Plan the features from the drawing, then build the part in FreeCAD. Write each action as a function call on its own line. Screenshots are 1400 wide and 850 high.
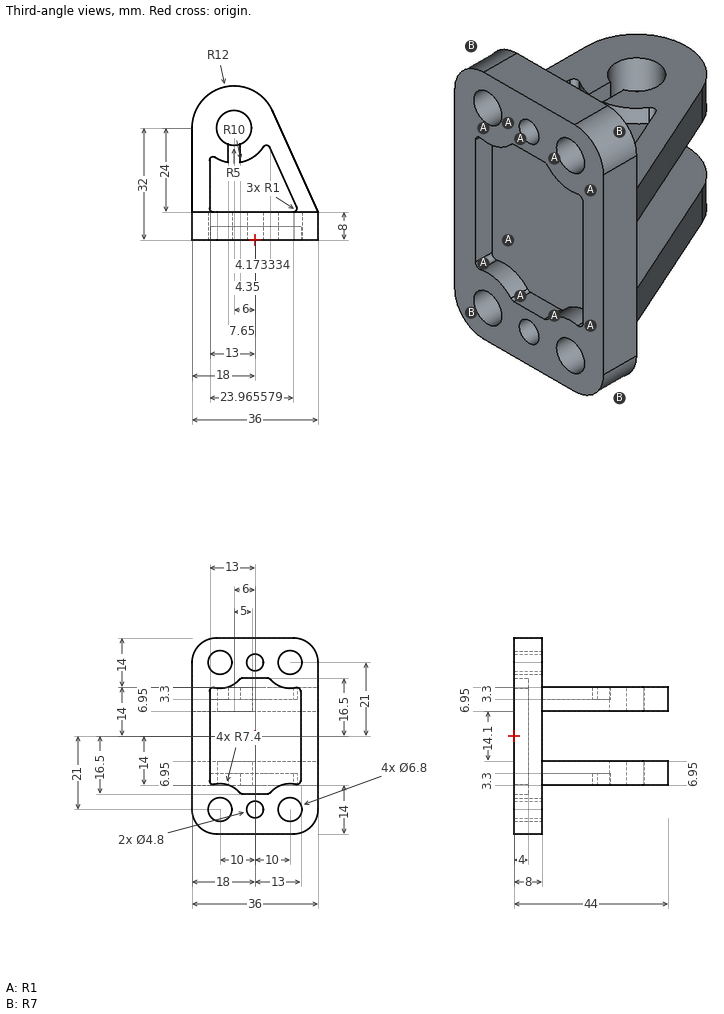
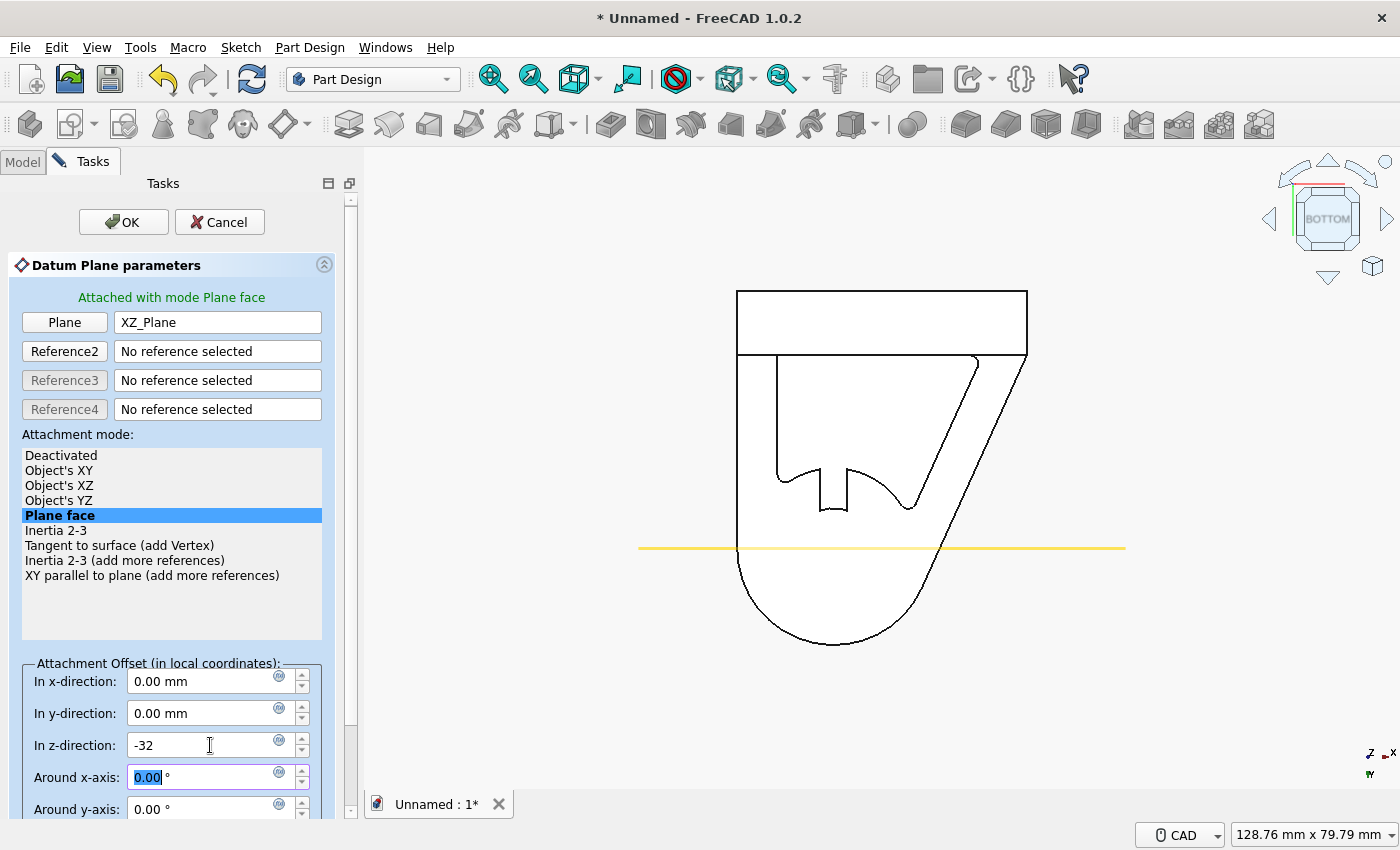
click(124, 222)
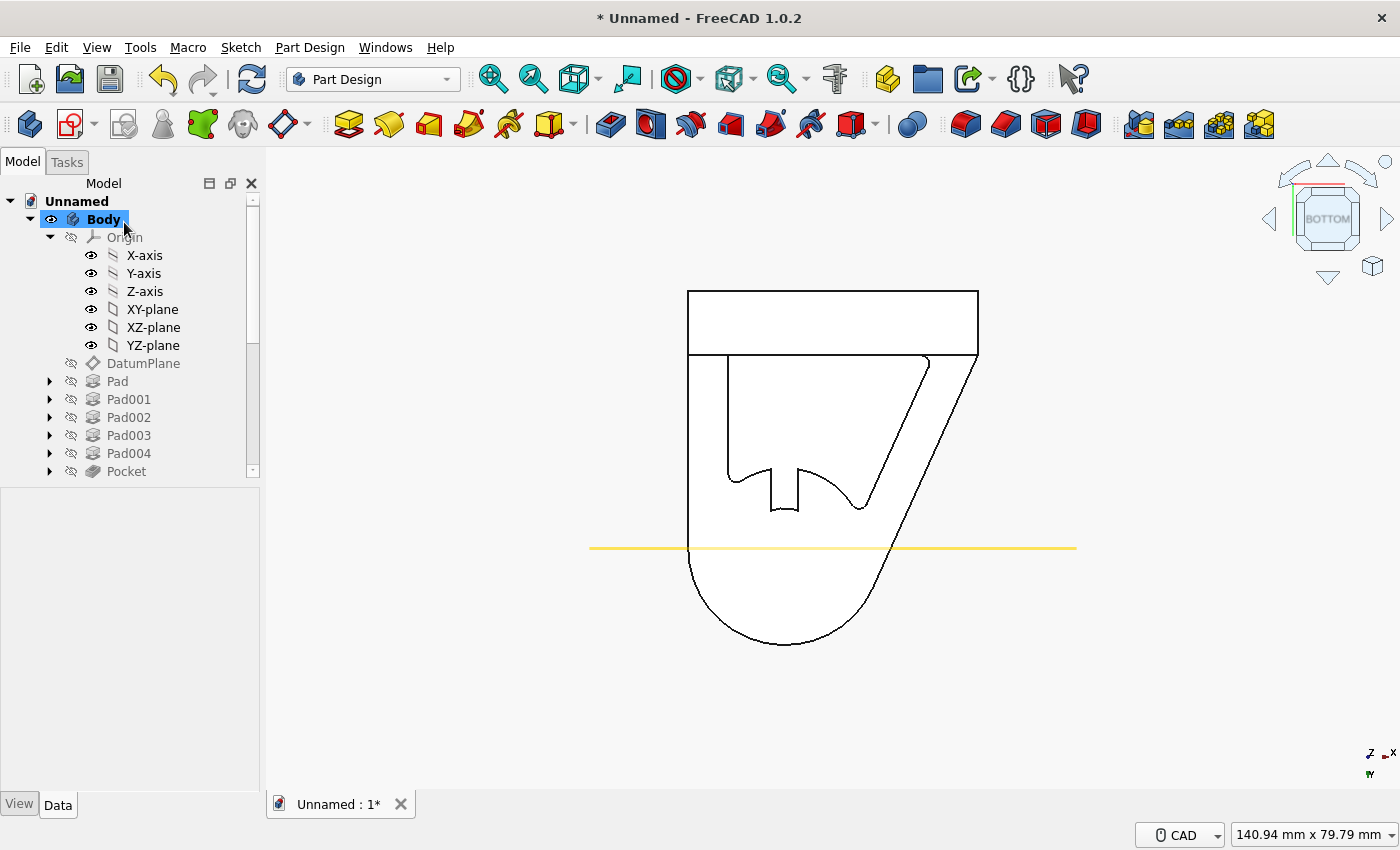
scroll(100, 341, down, 3)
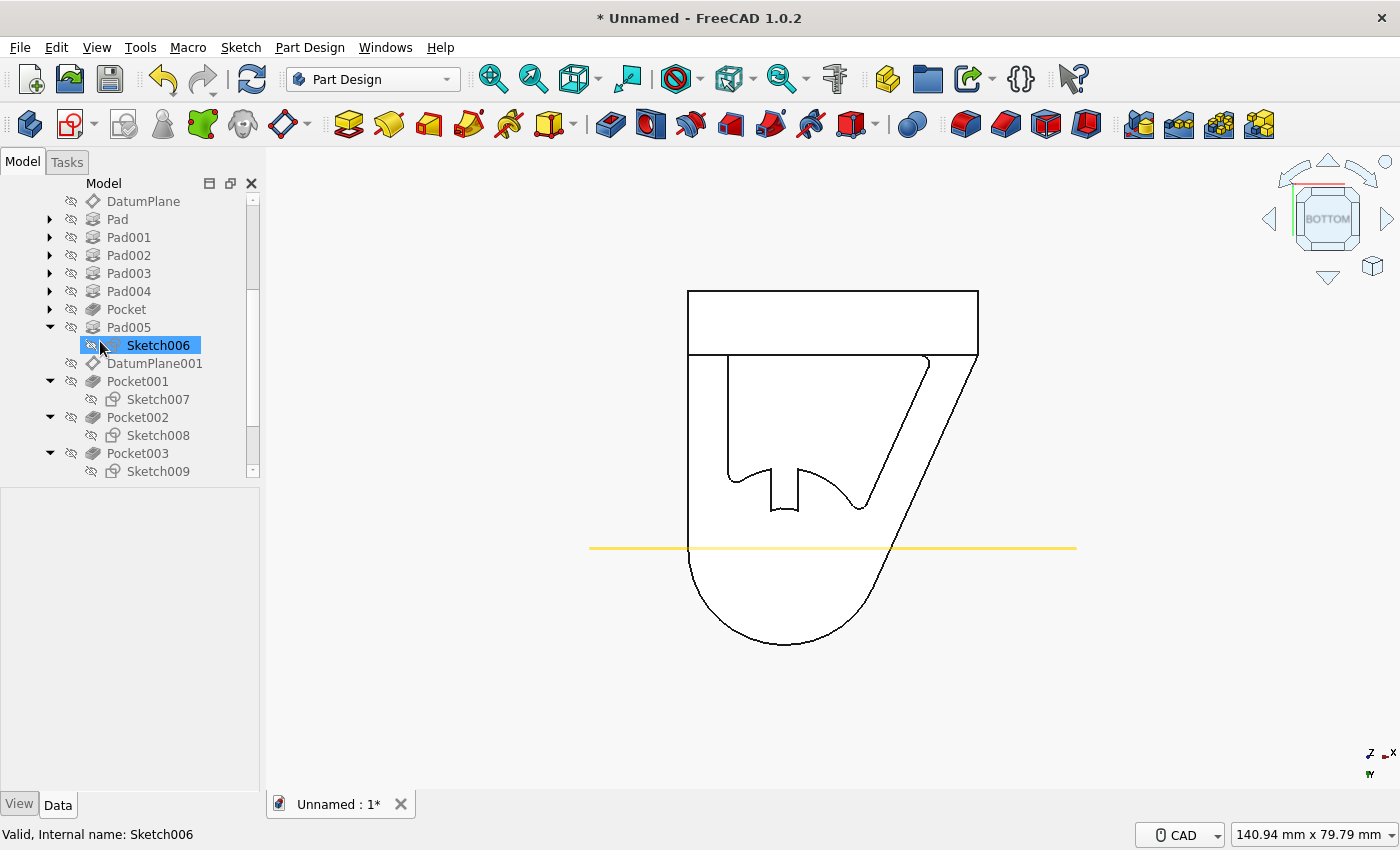
scroll(140, 341, up, 15)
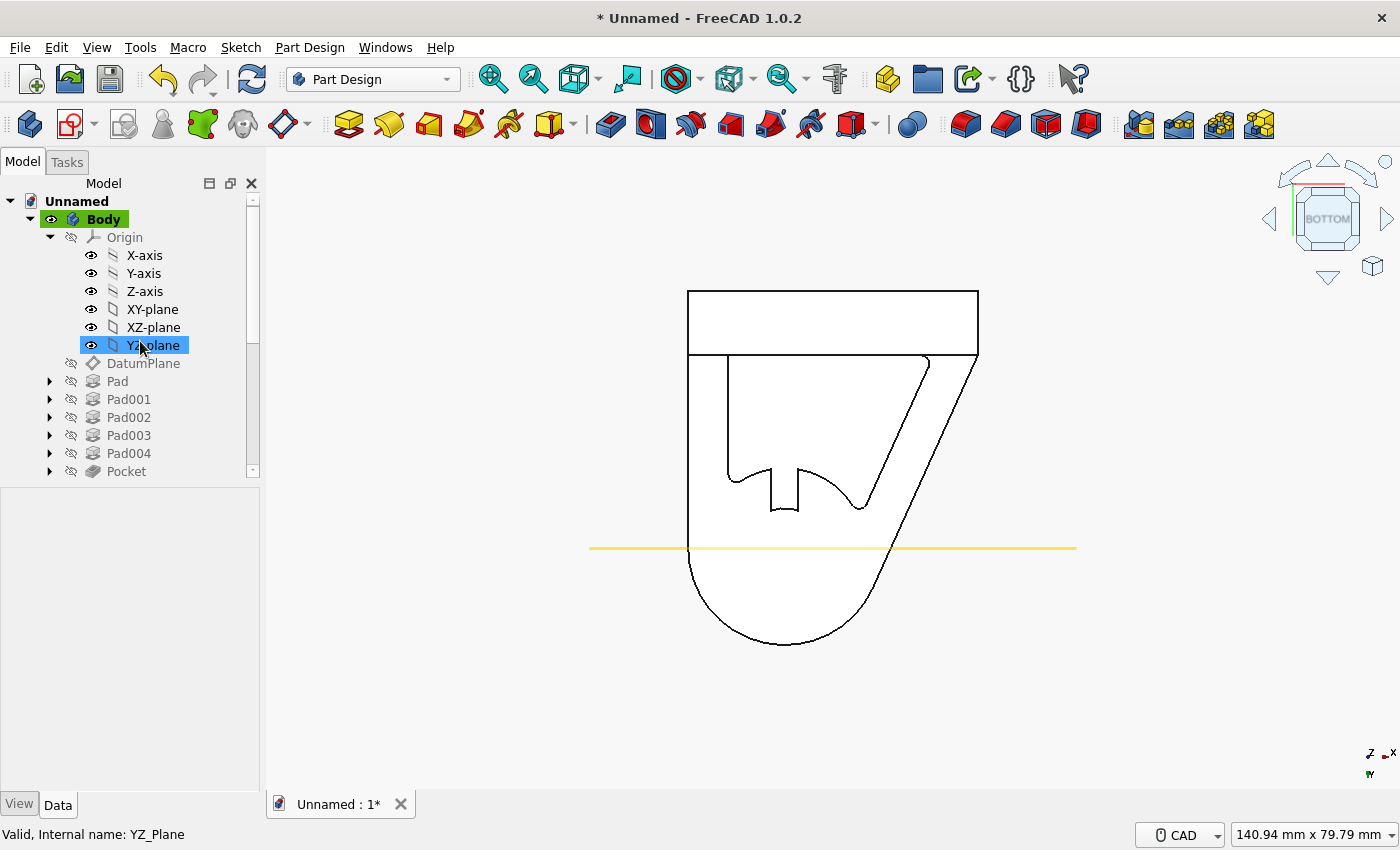
scroll(100, 341, down, 6)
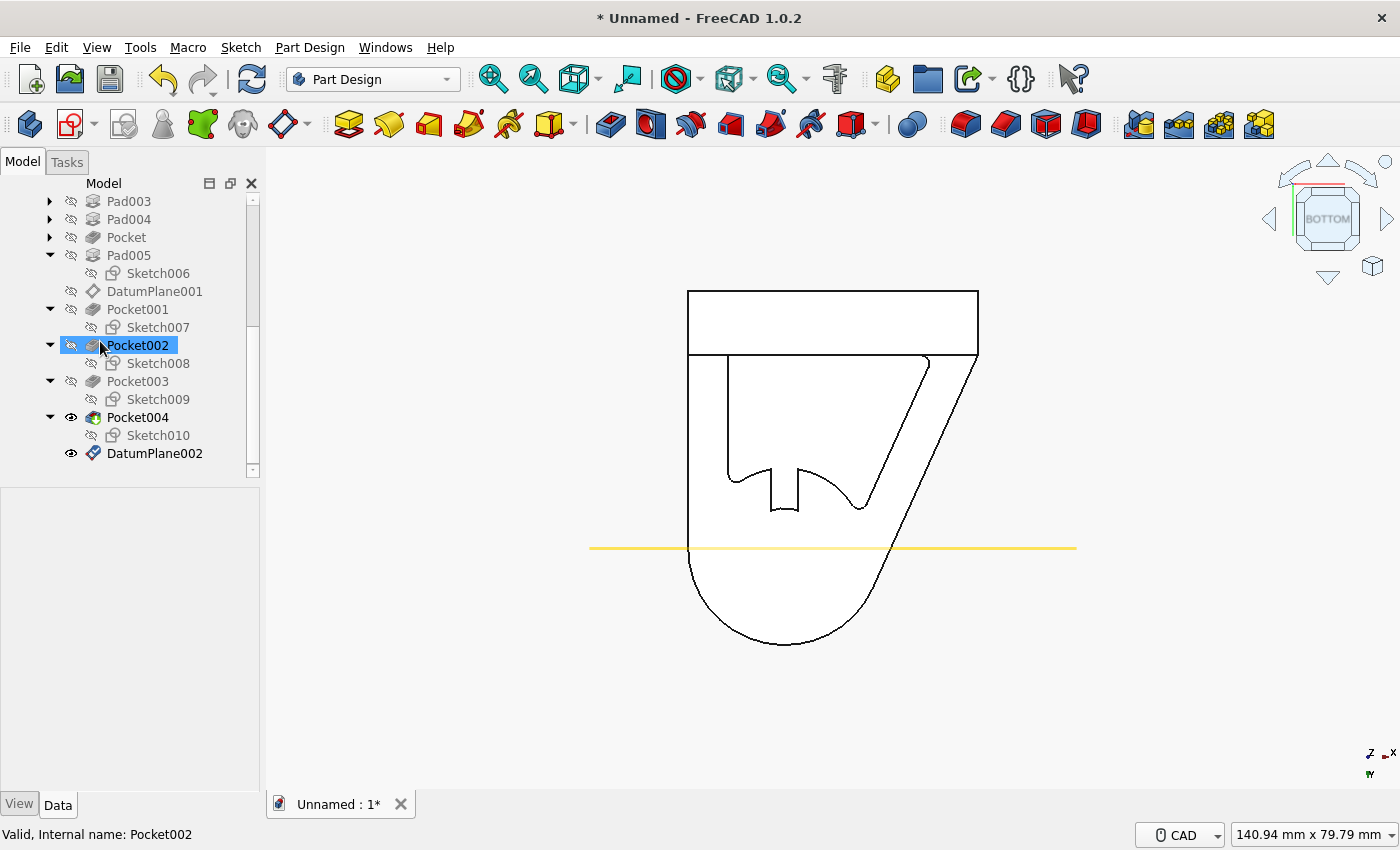
click(116, 453)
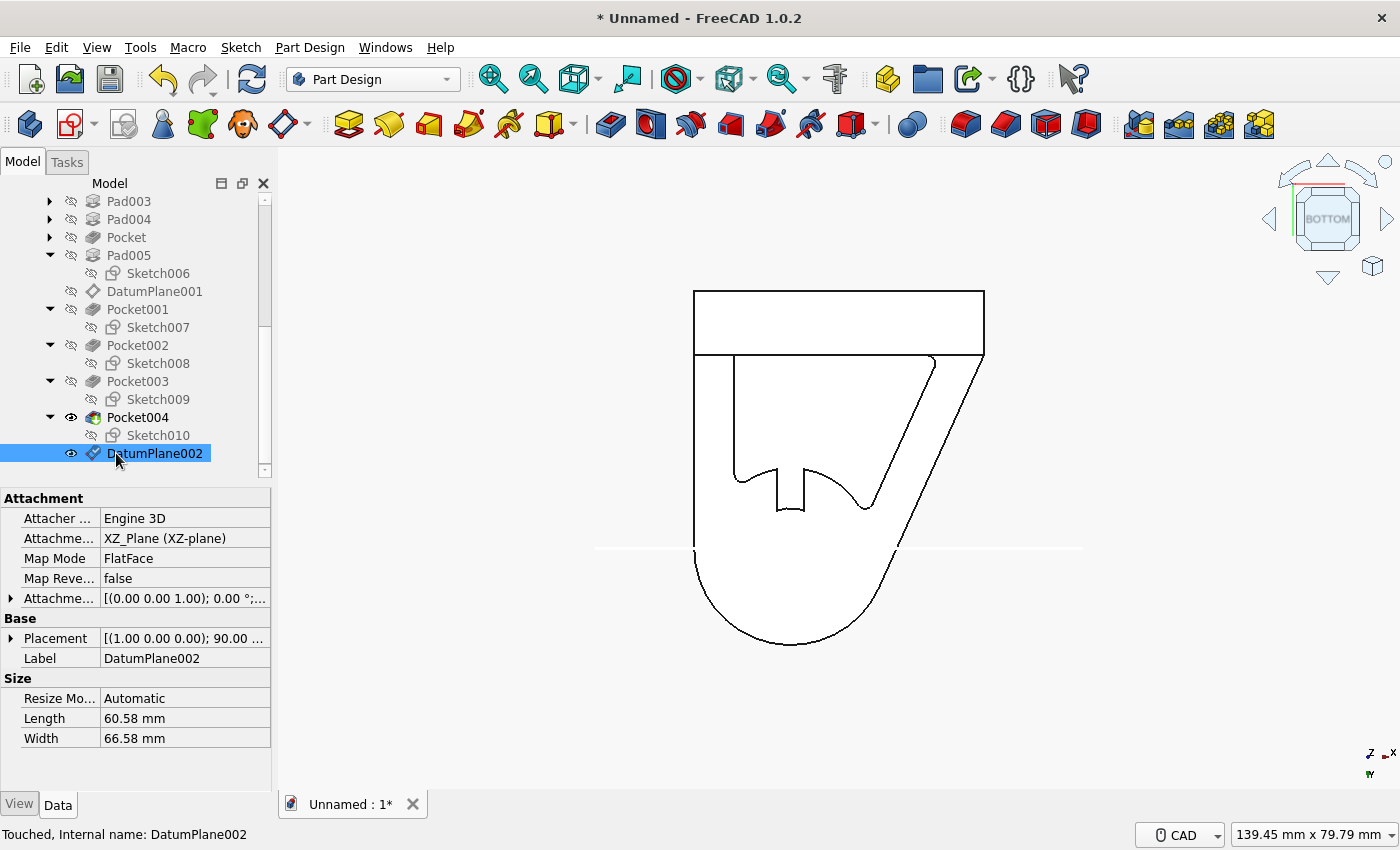
click(70, 124)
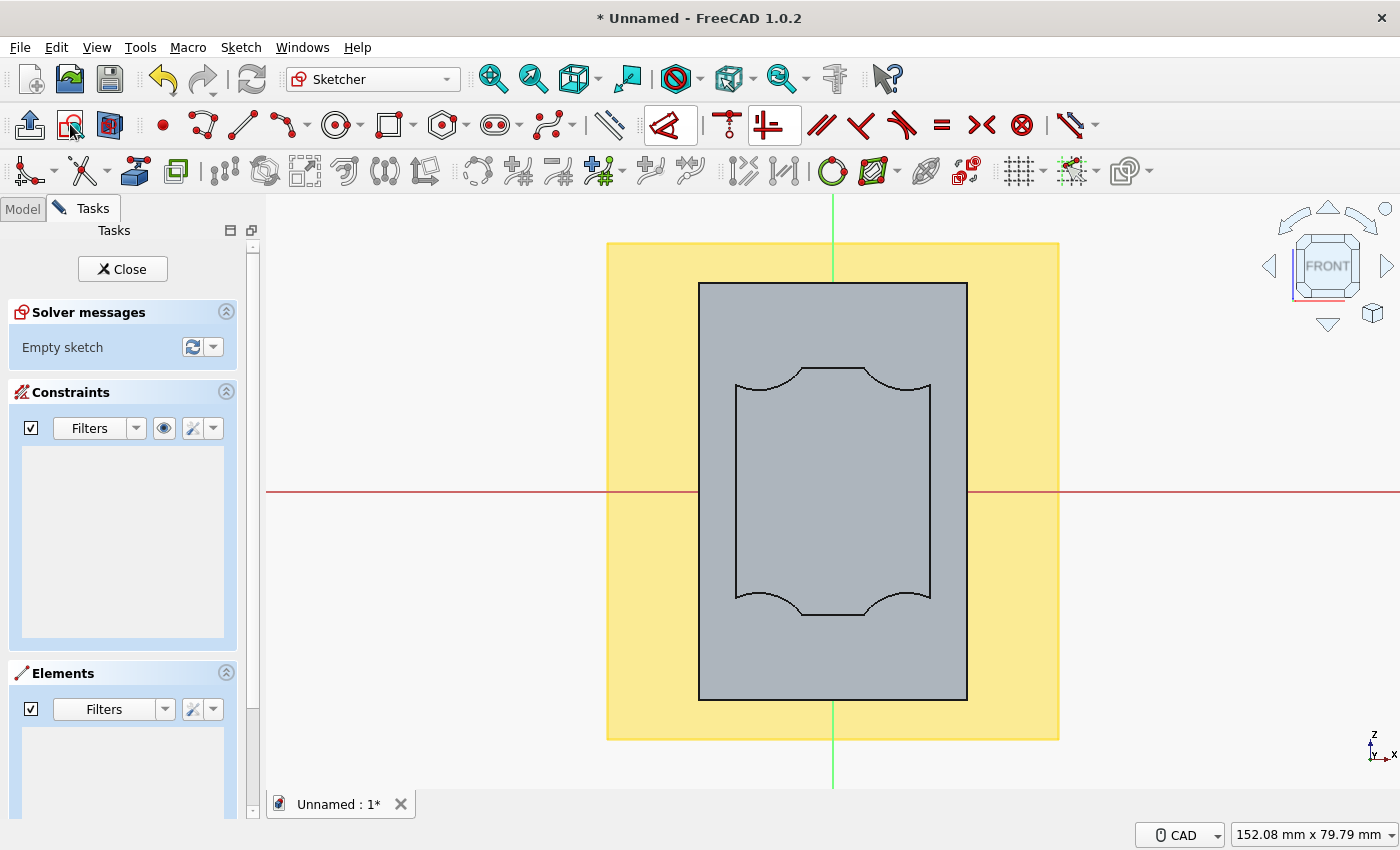
key(q)
key(s)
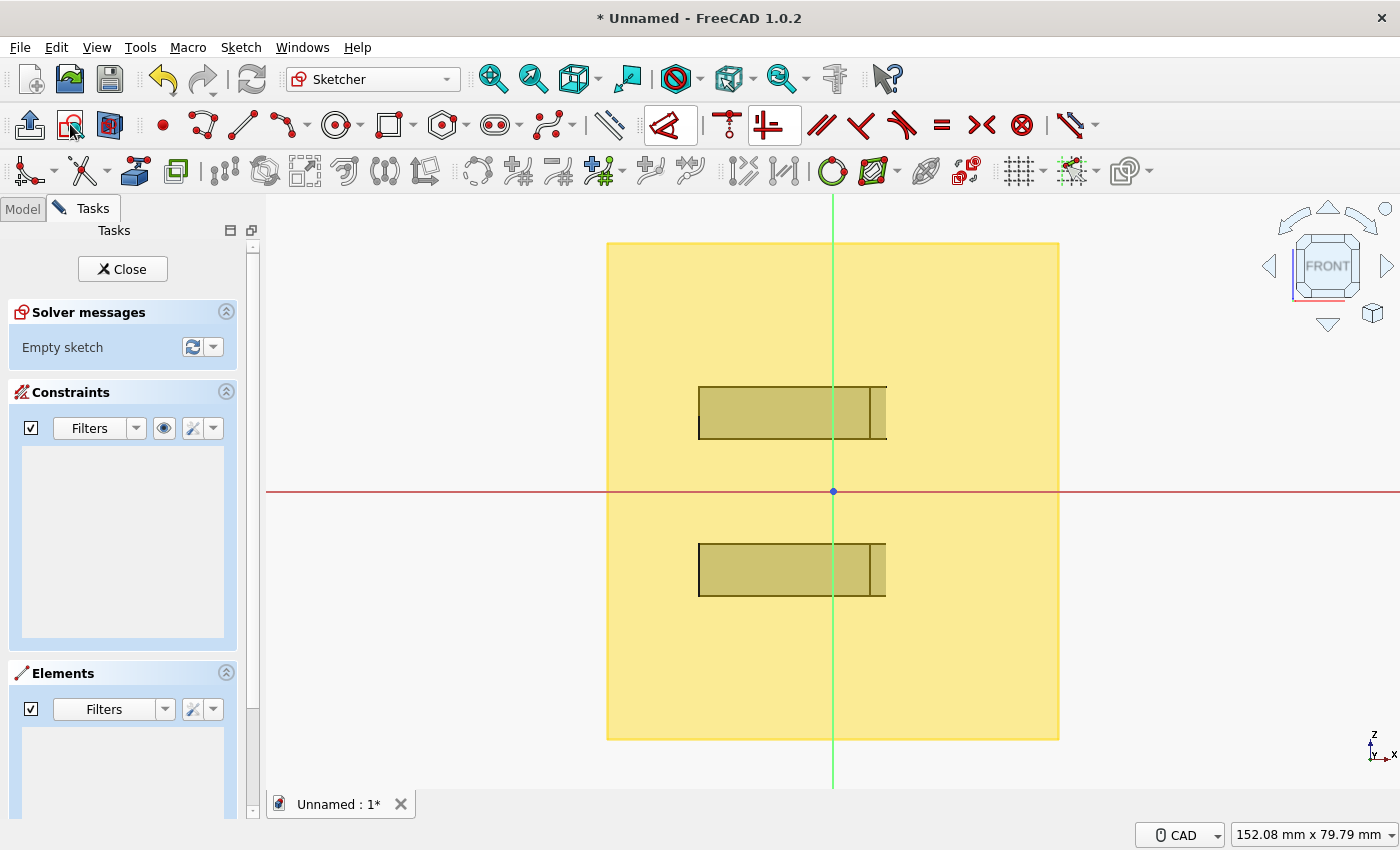
scroll(831, 402, up, 6)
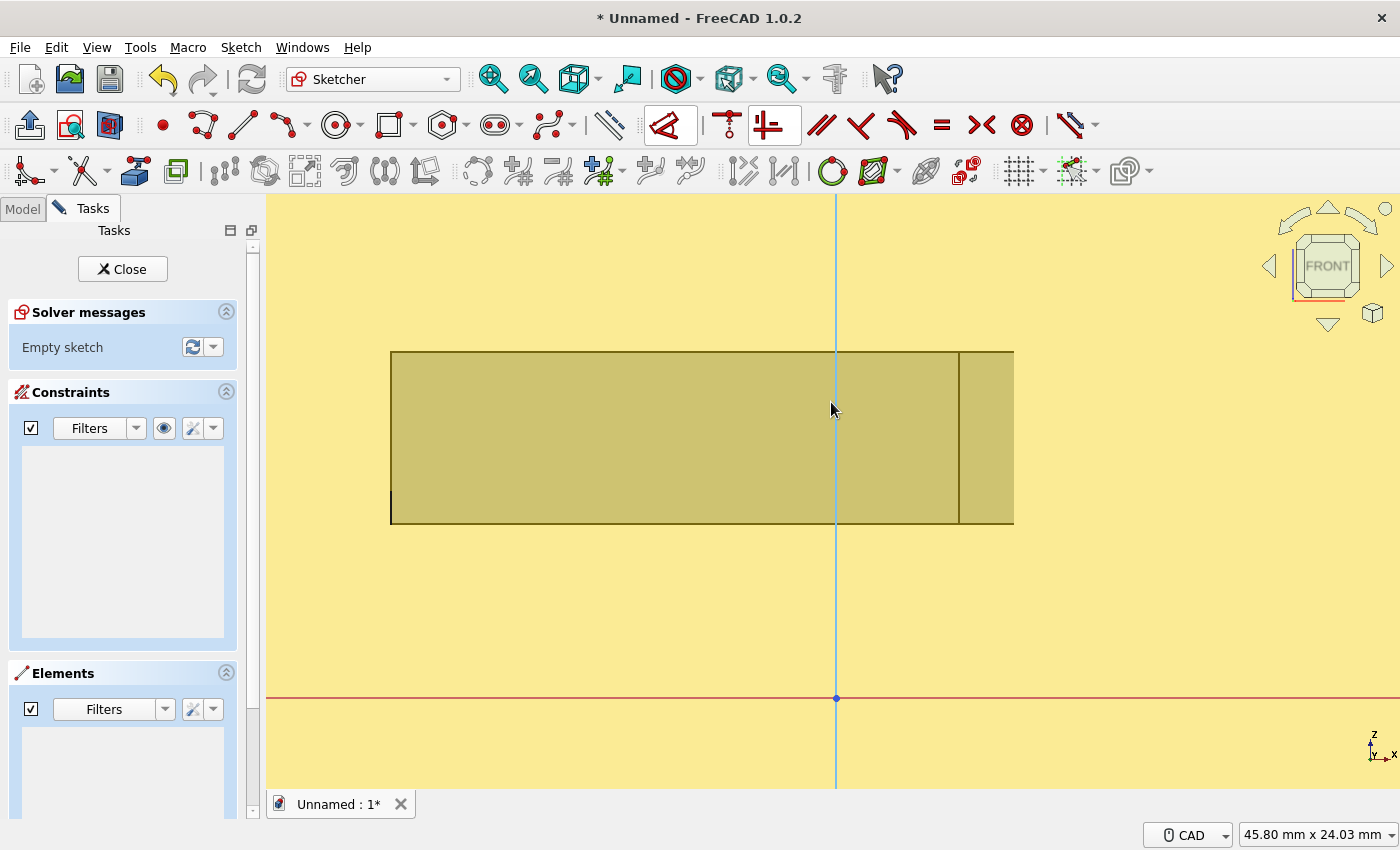
key(g)
key(r)